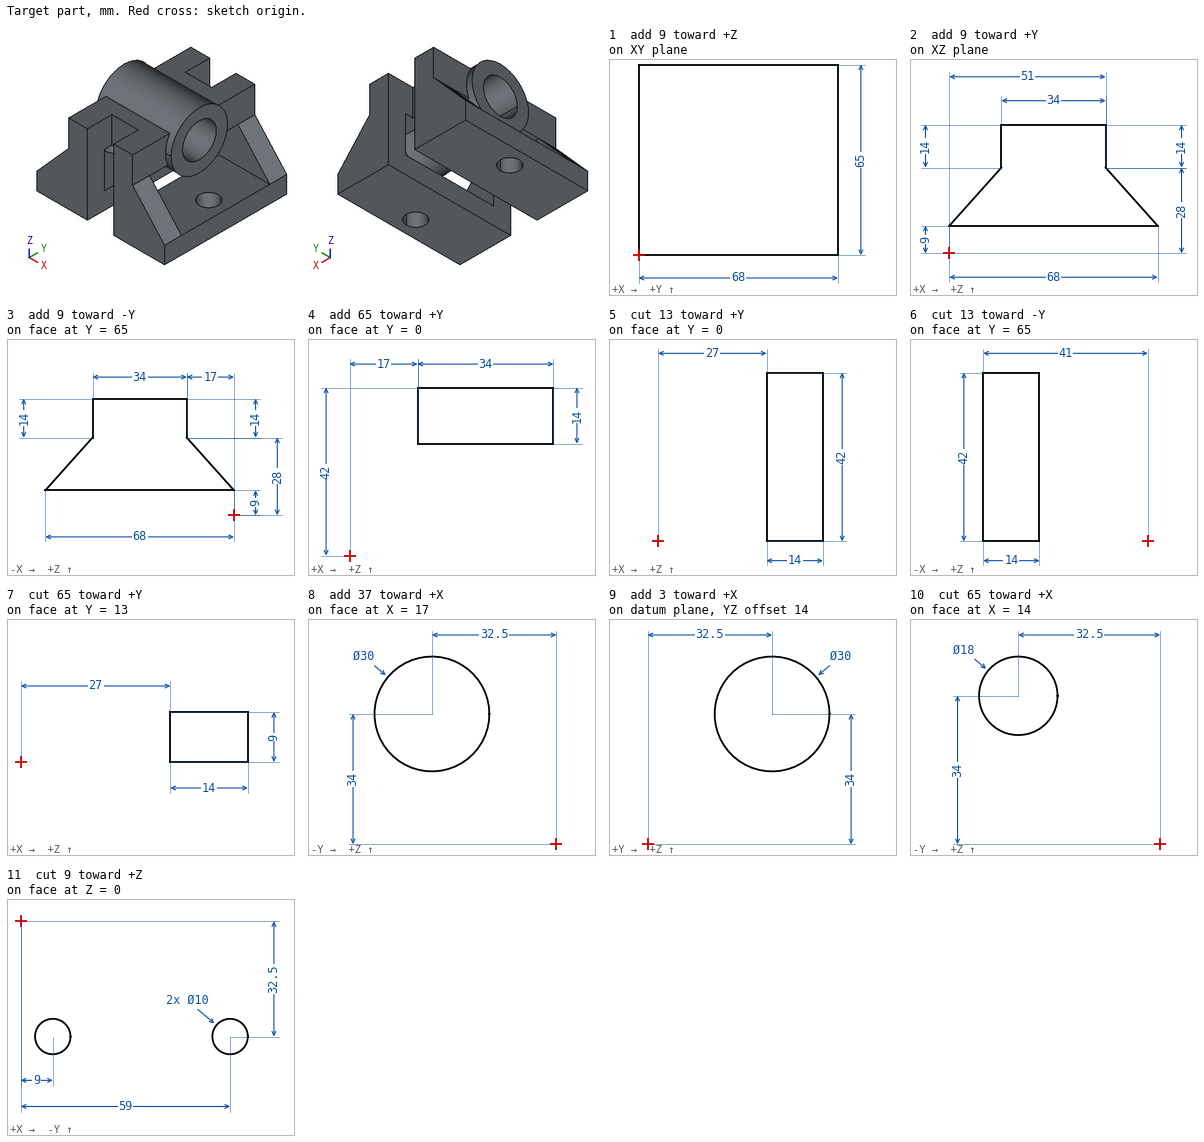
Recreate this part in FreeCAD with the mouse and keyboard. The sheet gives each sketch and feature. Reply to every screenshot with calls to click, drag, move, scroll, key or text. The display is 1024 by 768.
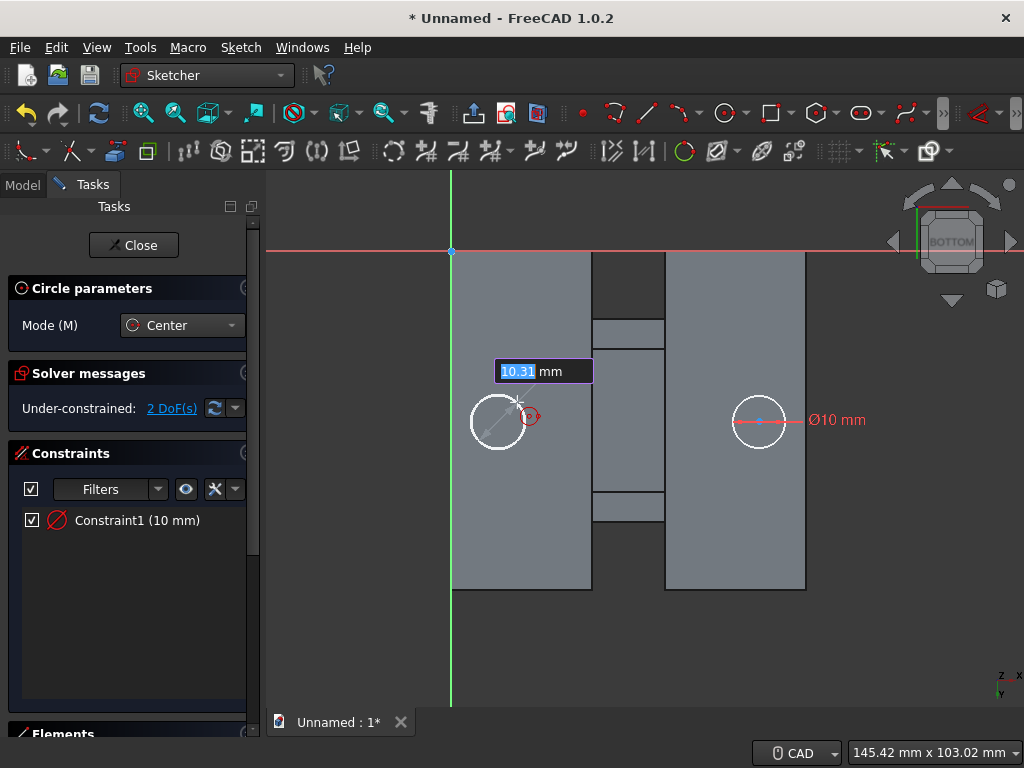
text(10)
key(Return)
key(Escape)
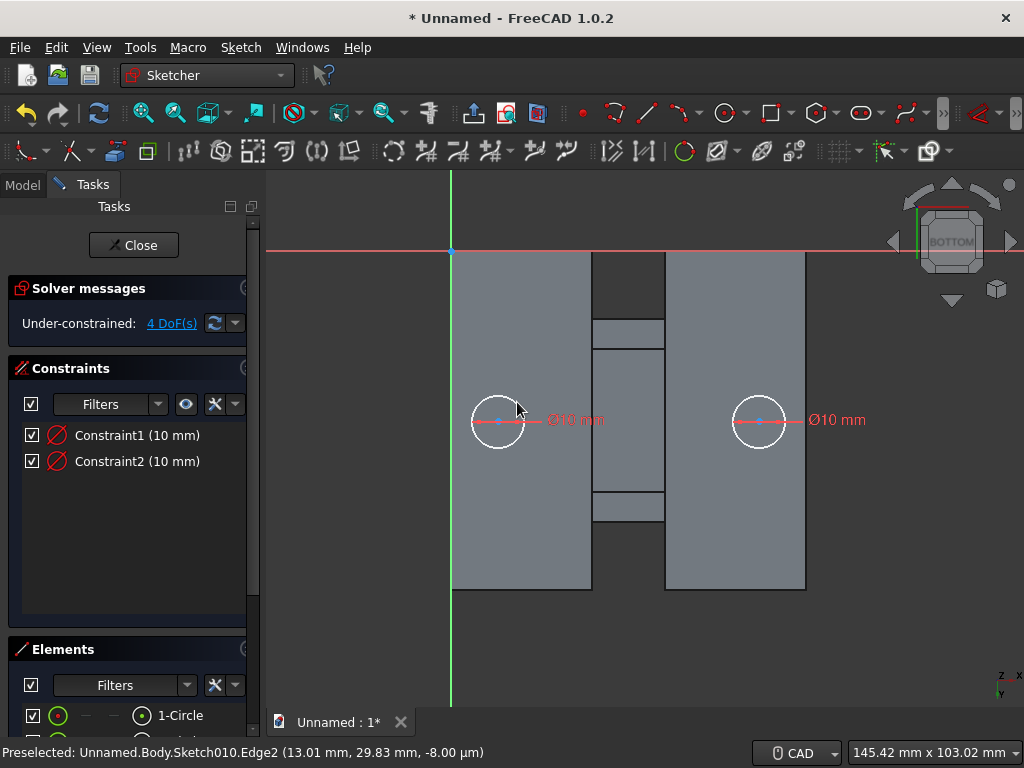
click(759, 422)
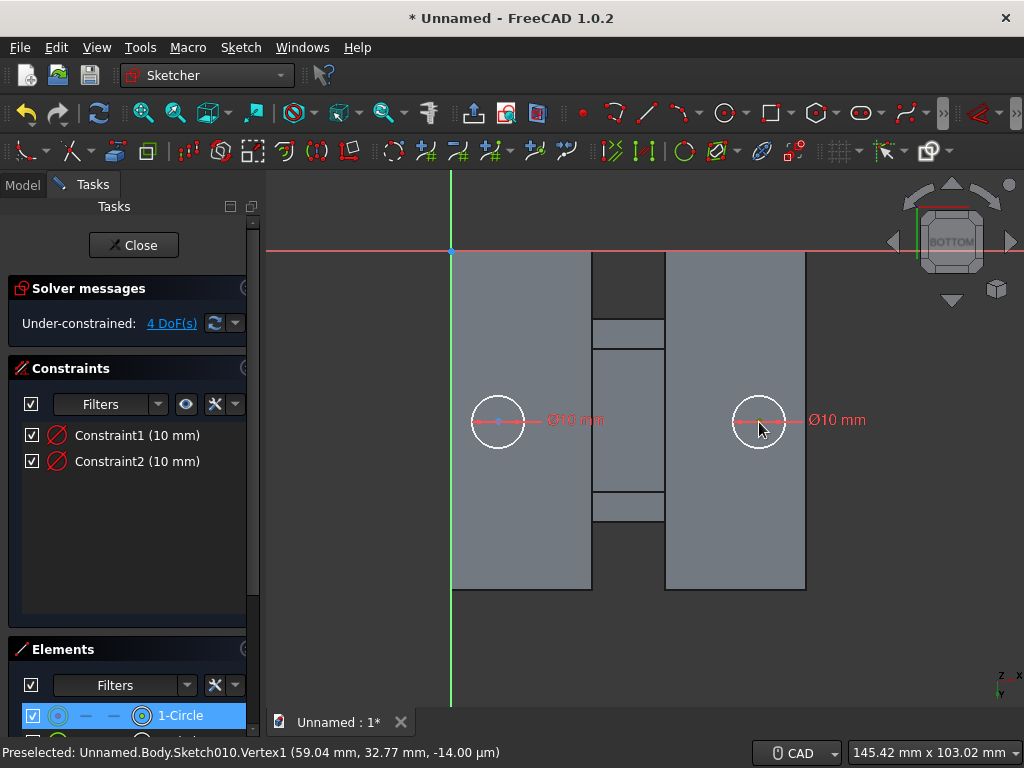
click(498, 422)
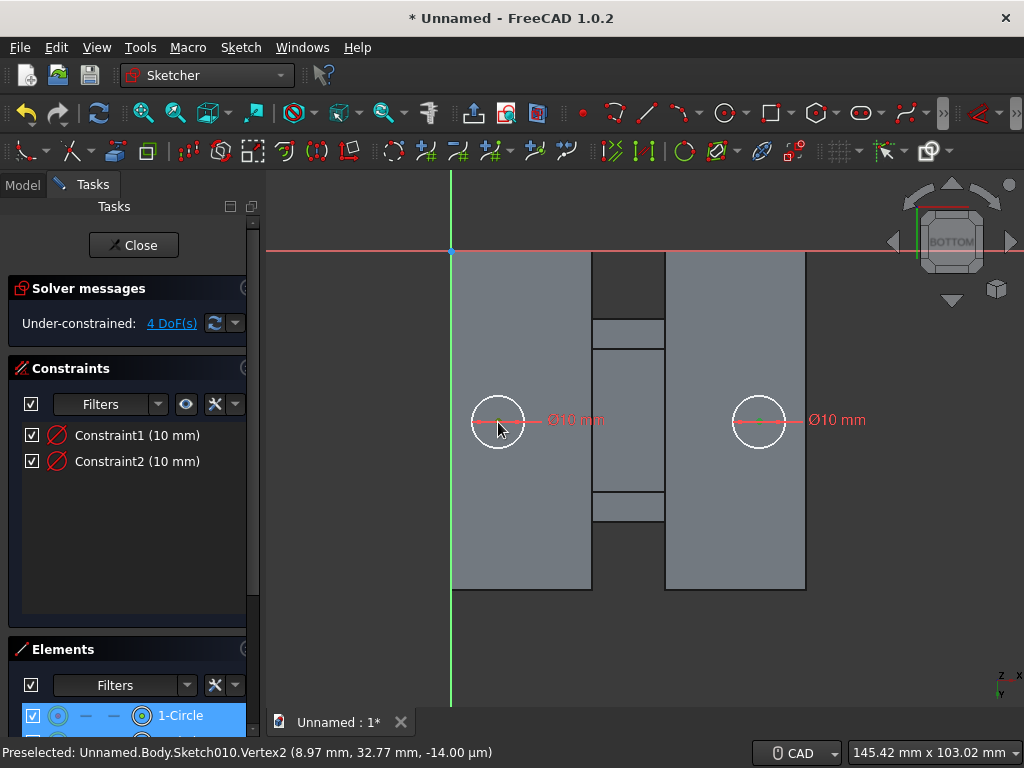
key(h)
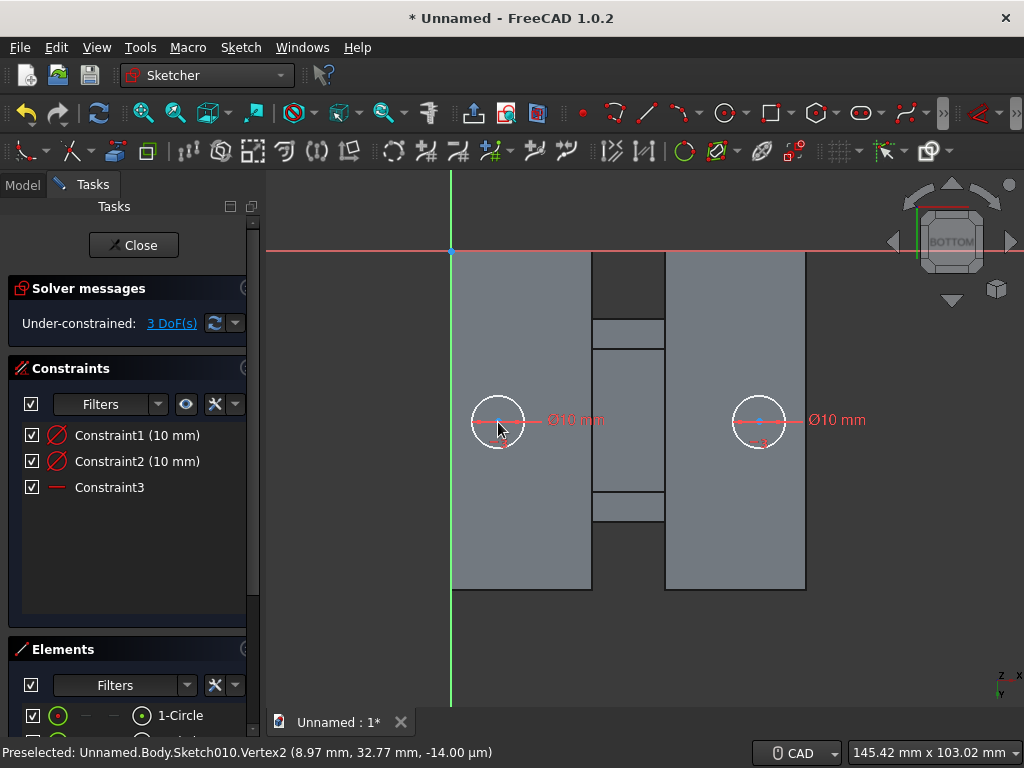
click(978, 114)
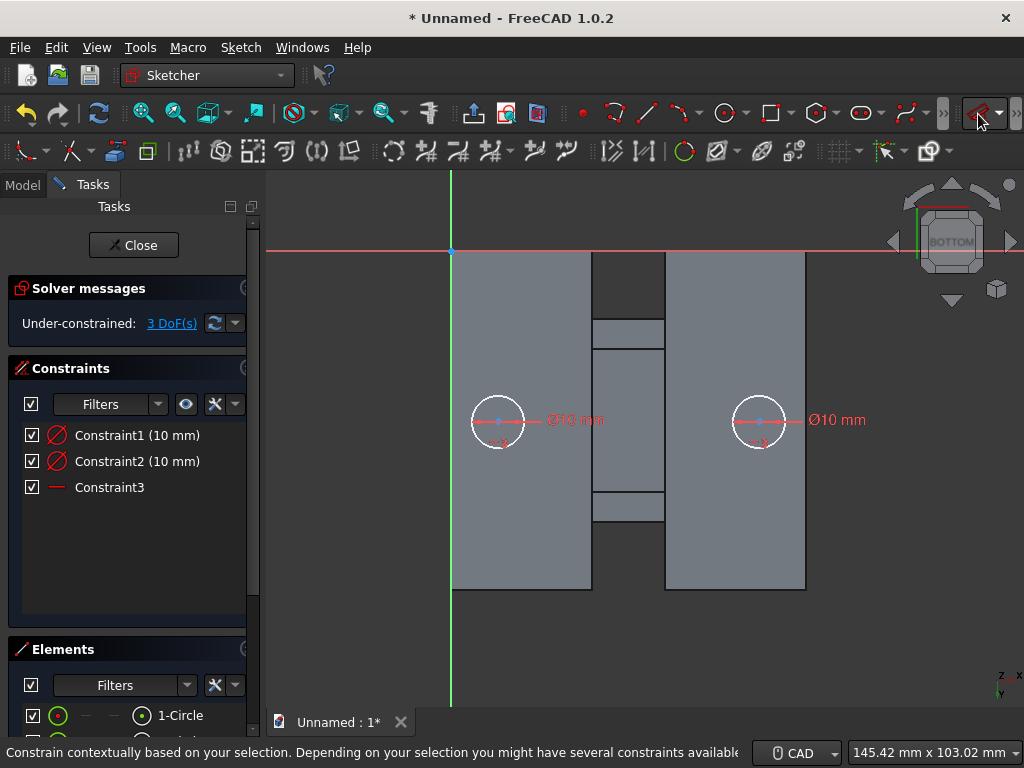
click(498, 422)
click(475, 217)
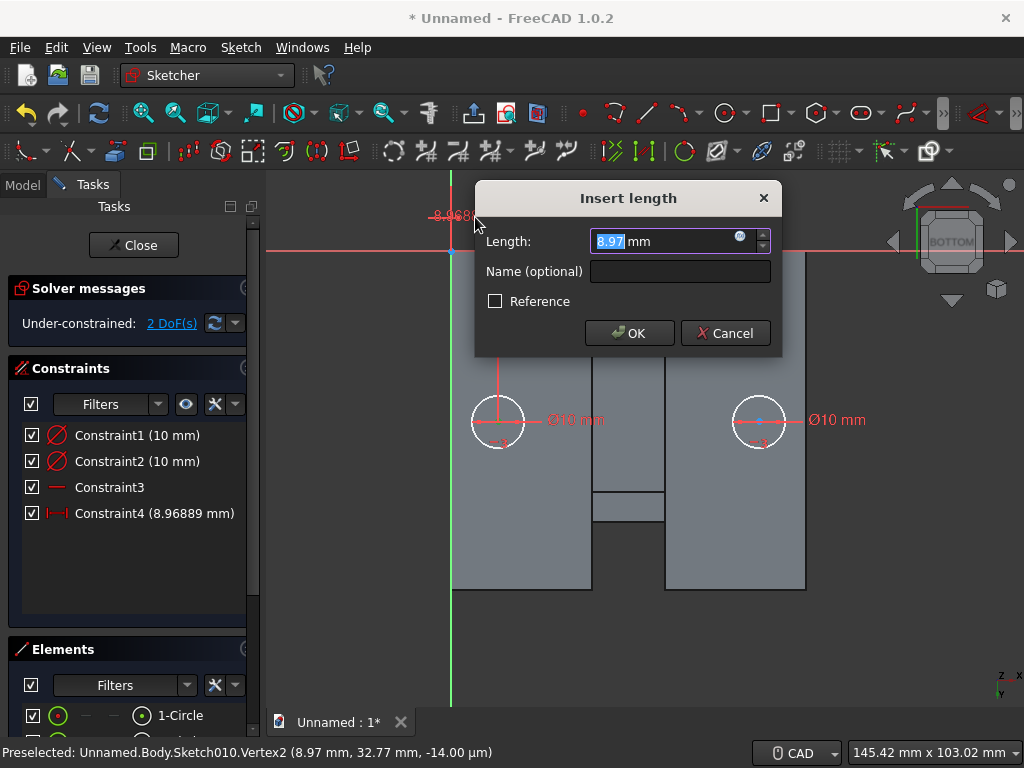
text(9)
key(Return)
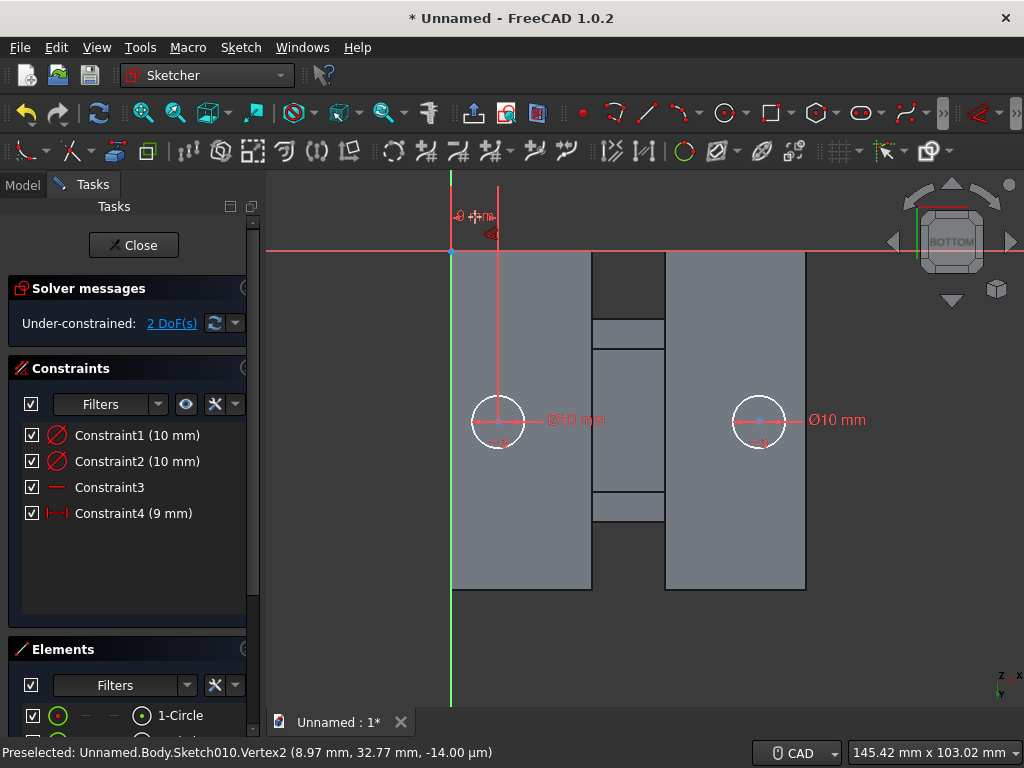
click(759, 422)
click(605, 217)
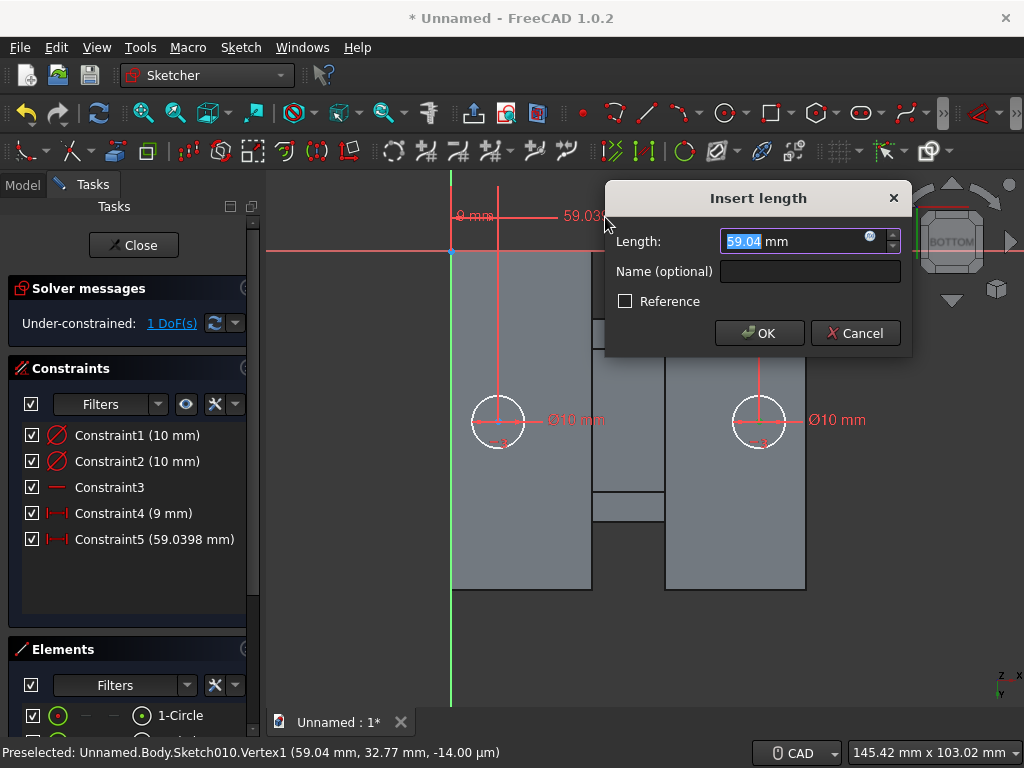
text(59)
key(Return)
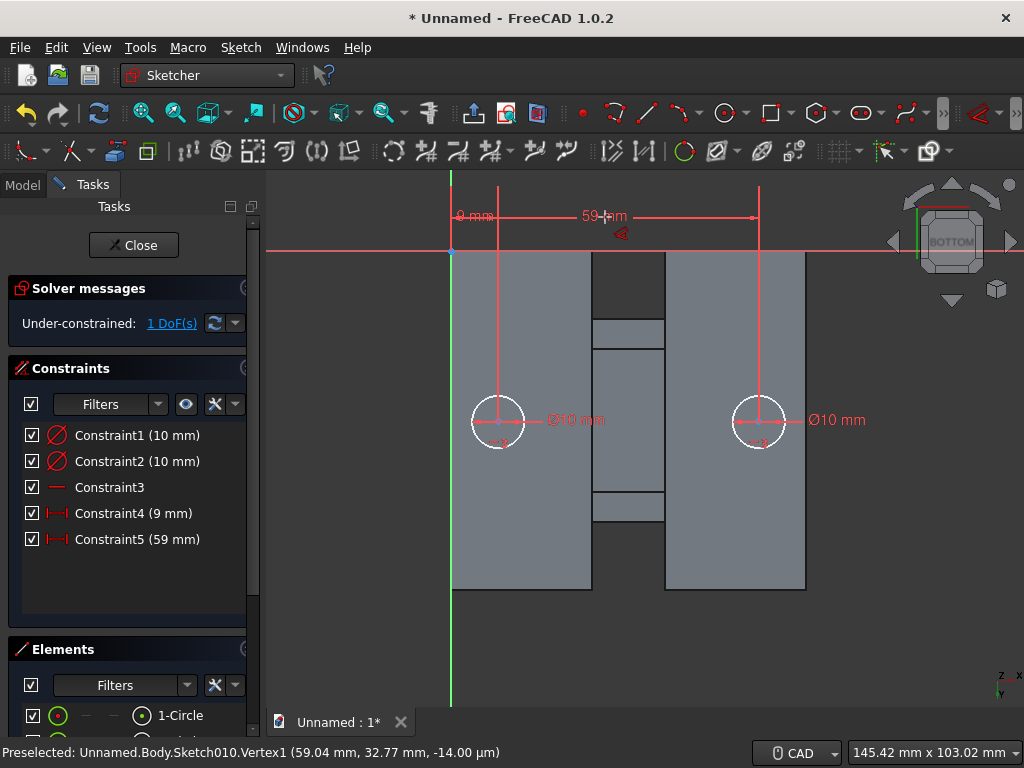
click(759, 422)
click(417, 337)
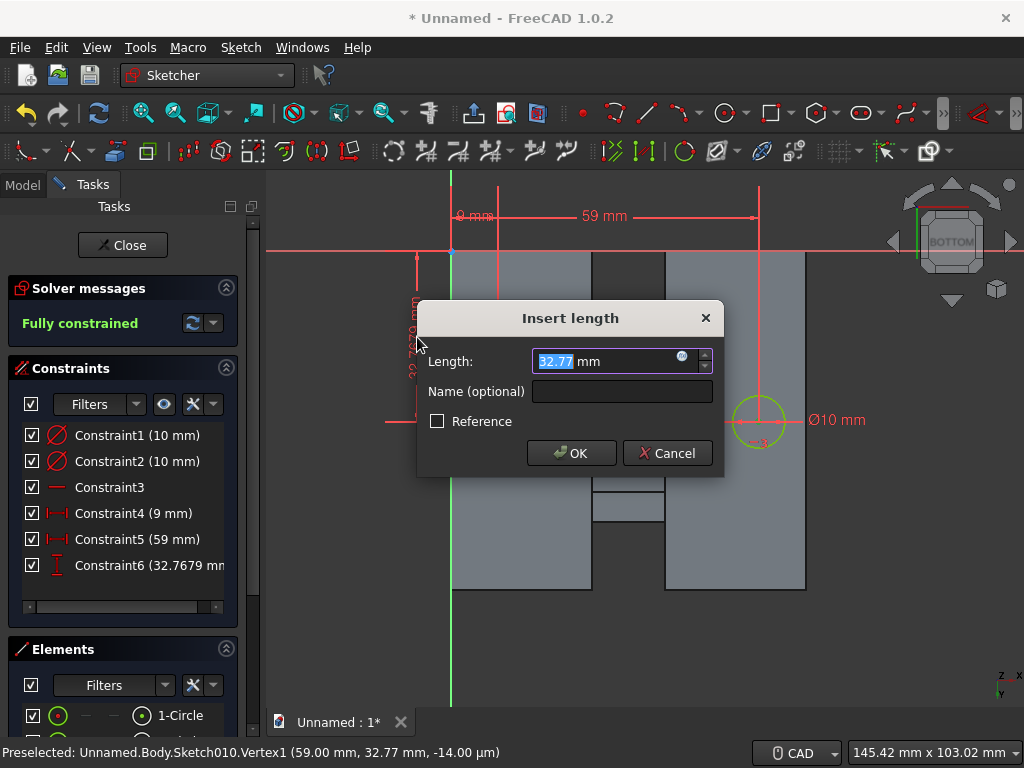
text(32.5)
key(Return)
key(Escape)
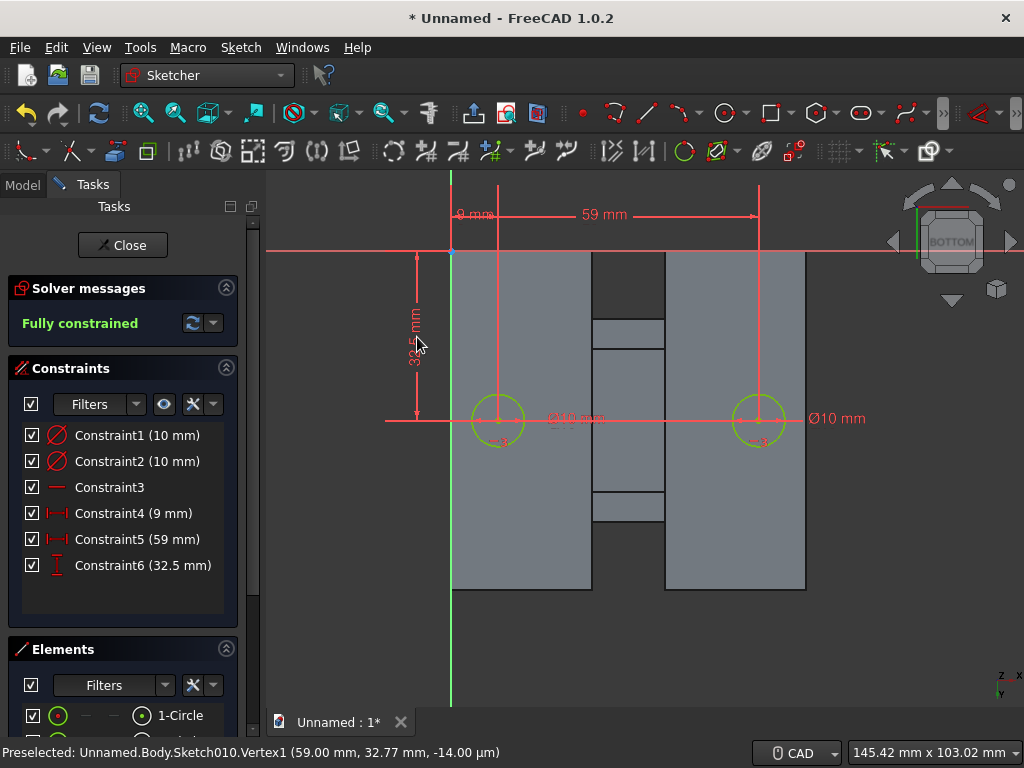
click(123, 245)